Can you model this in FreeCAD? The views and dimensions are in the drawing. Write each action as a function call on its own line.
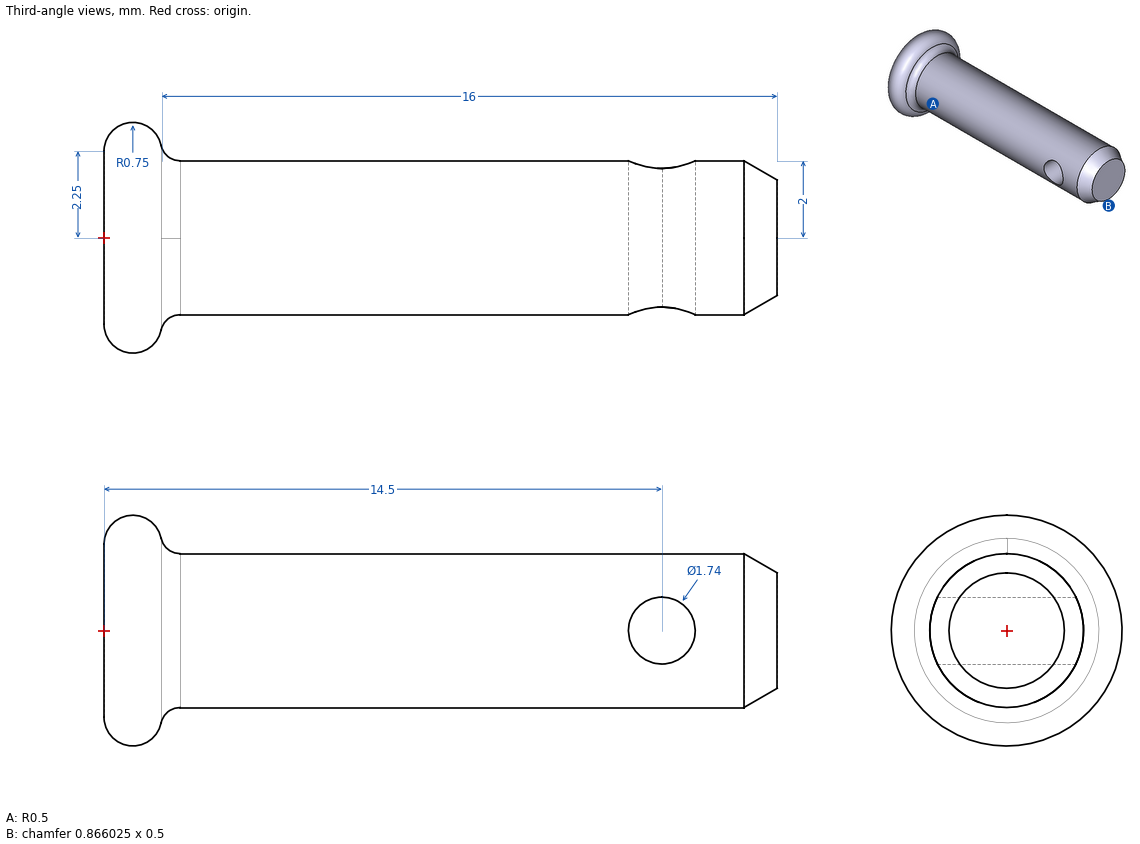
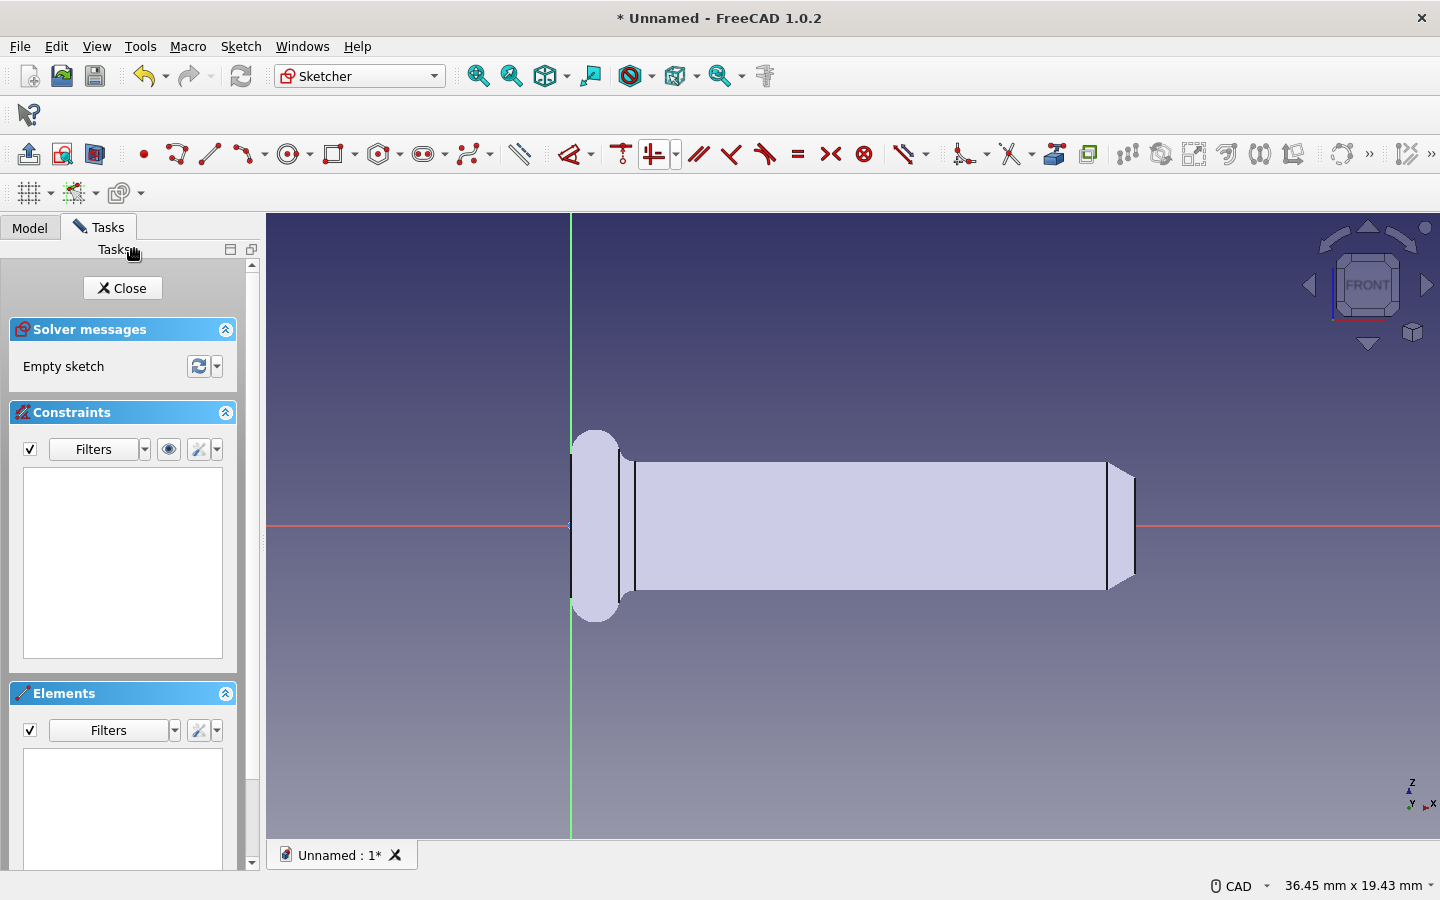
click(95, 154)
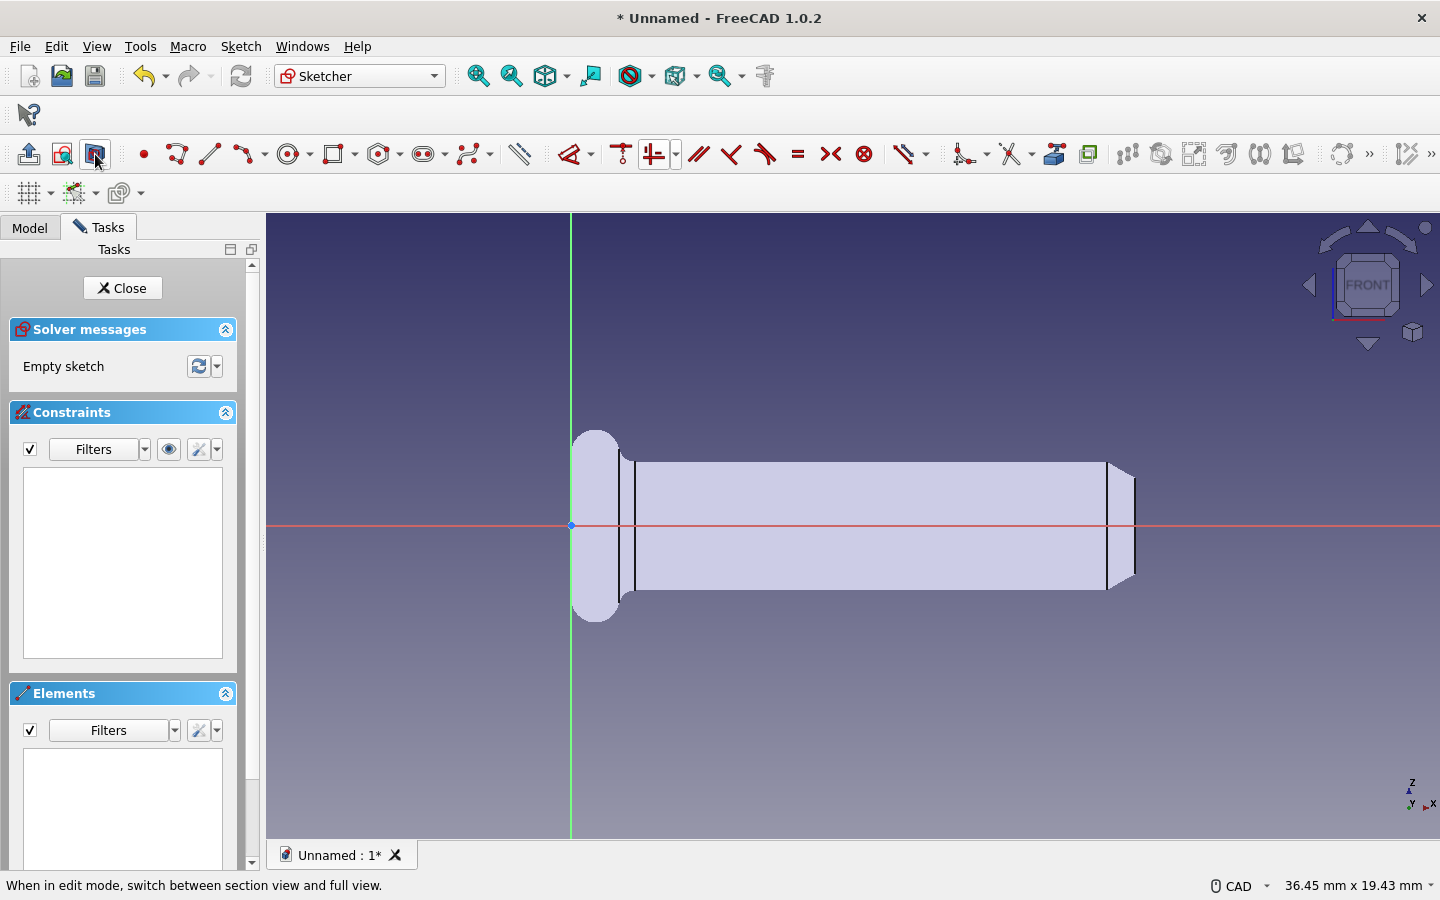
scroll(1078, 526, up, 10)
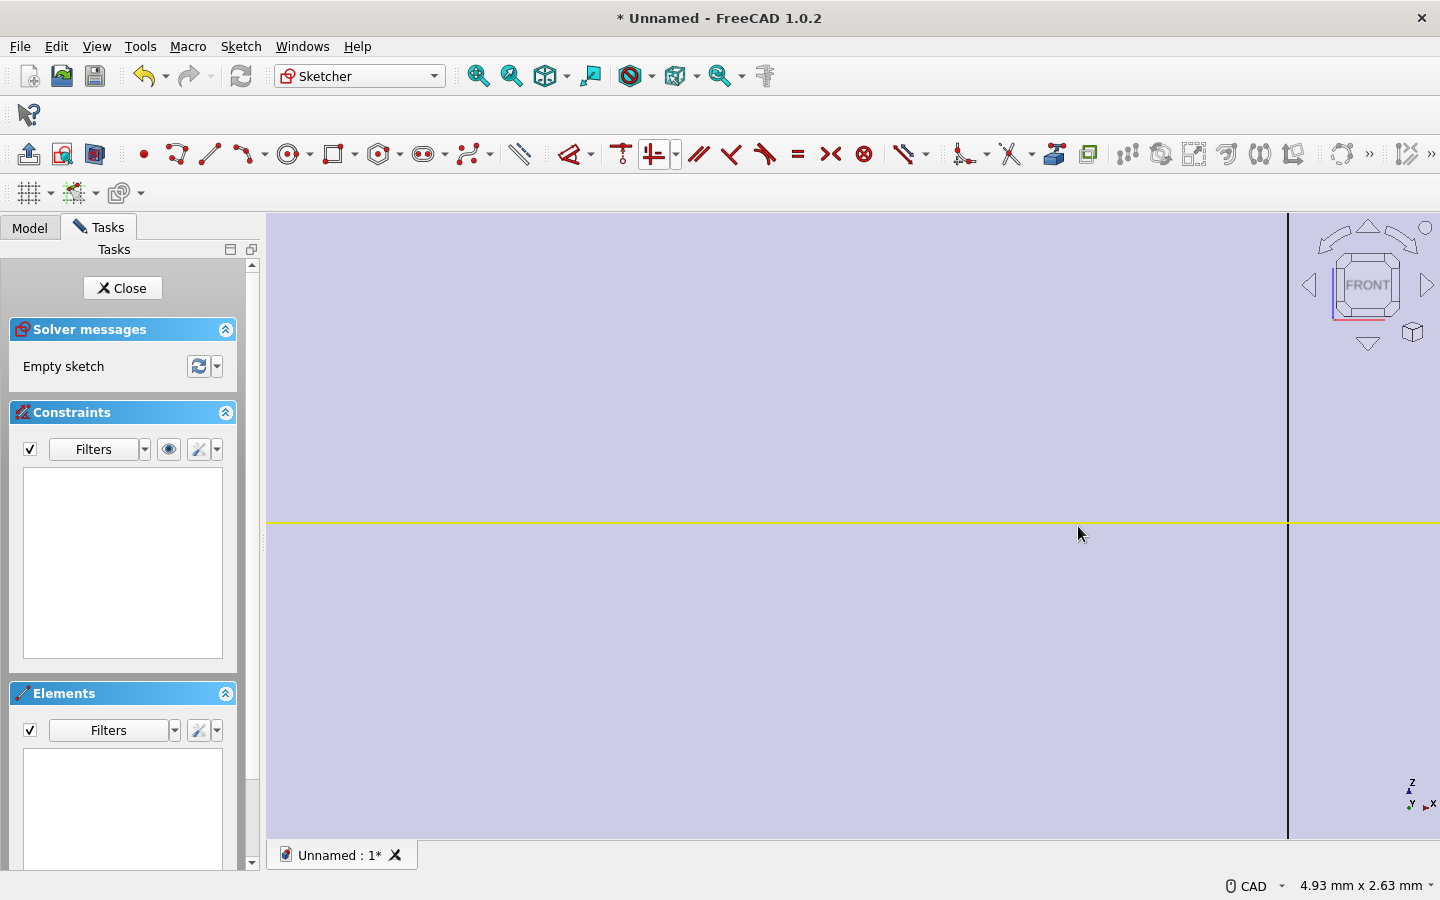
click(288, 154)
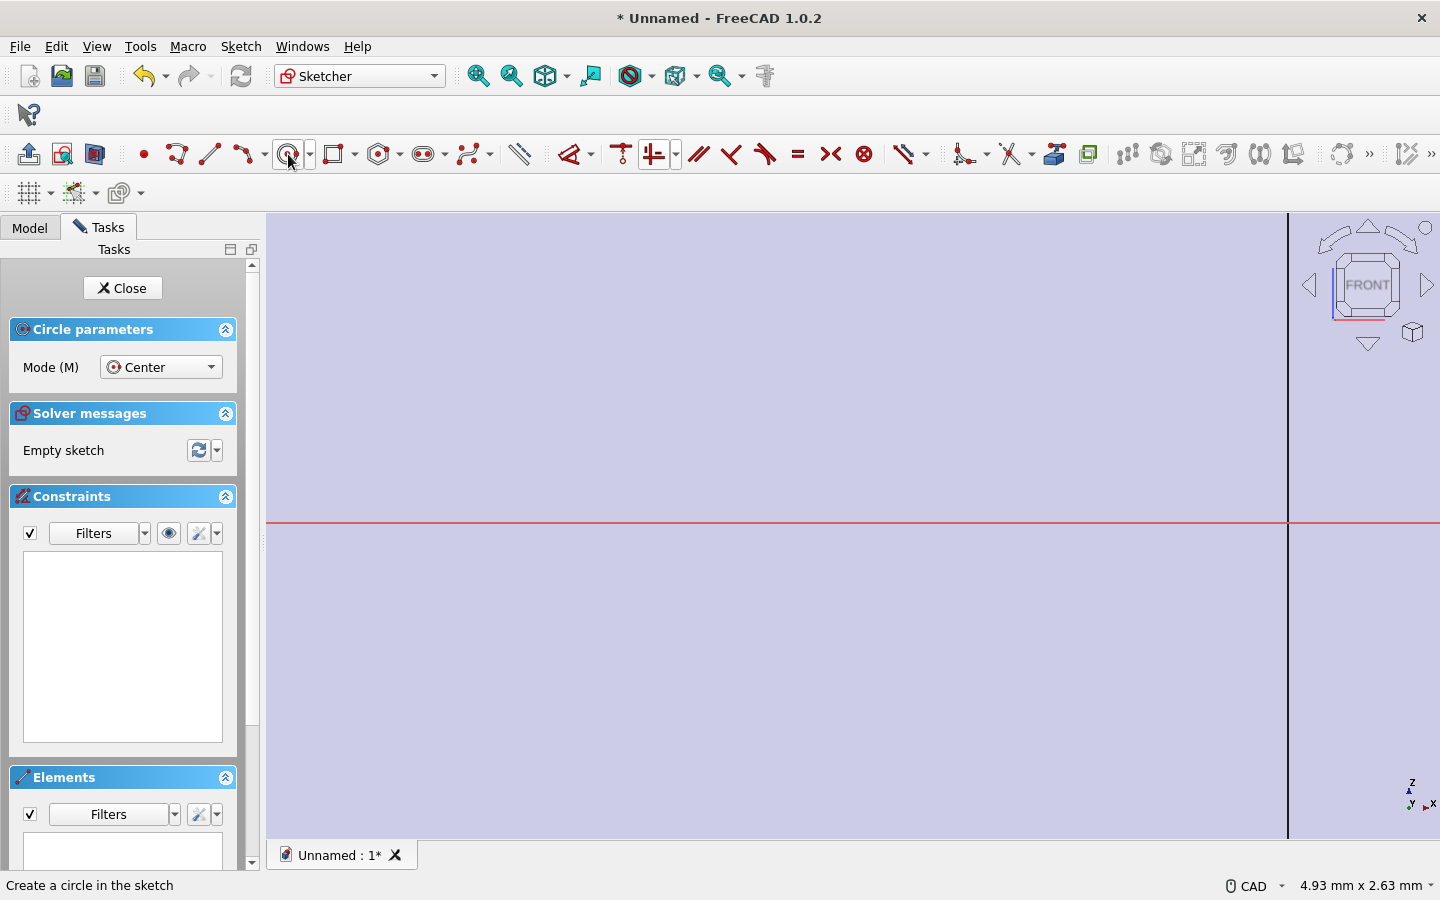
click(780, 523)
move(926, 376)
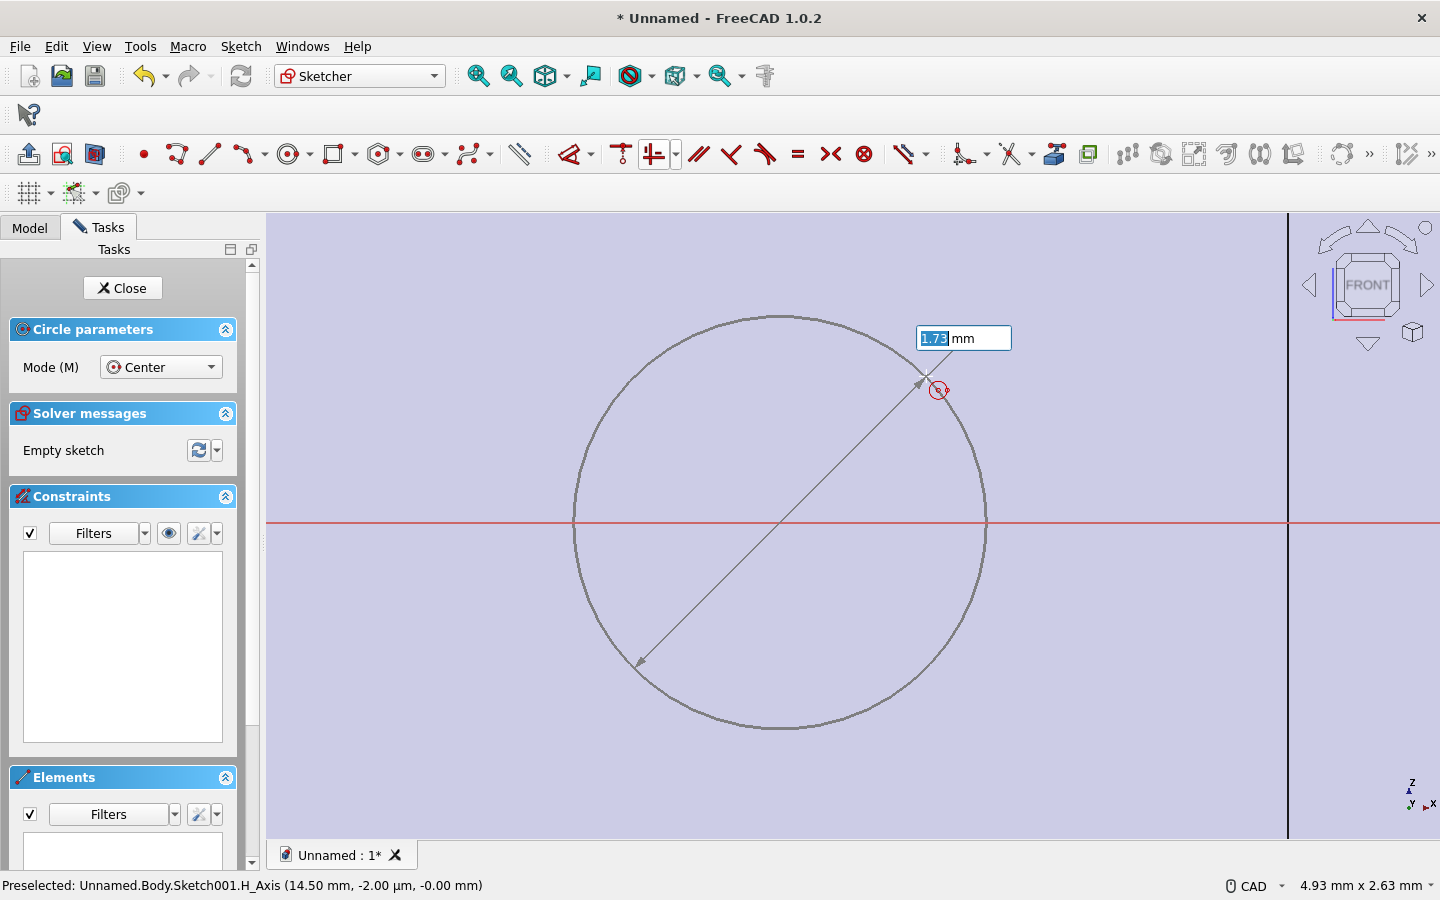
text(1.74)
key(Return)
key(Escape)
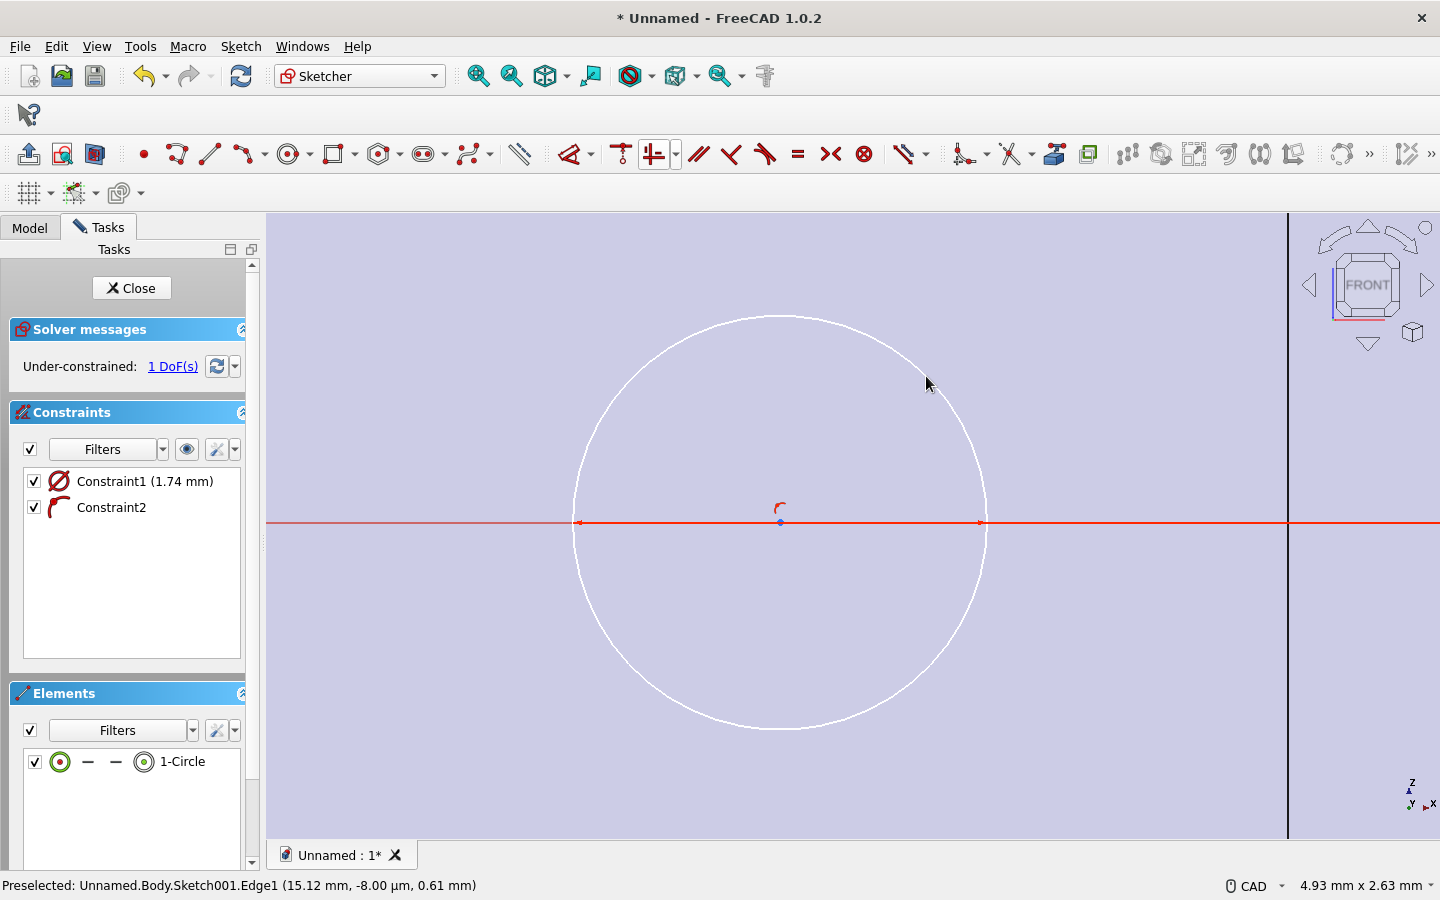
click(568, 154)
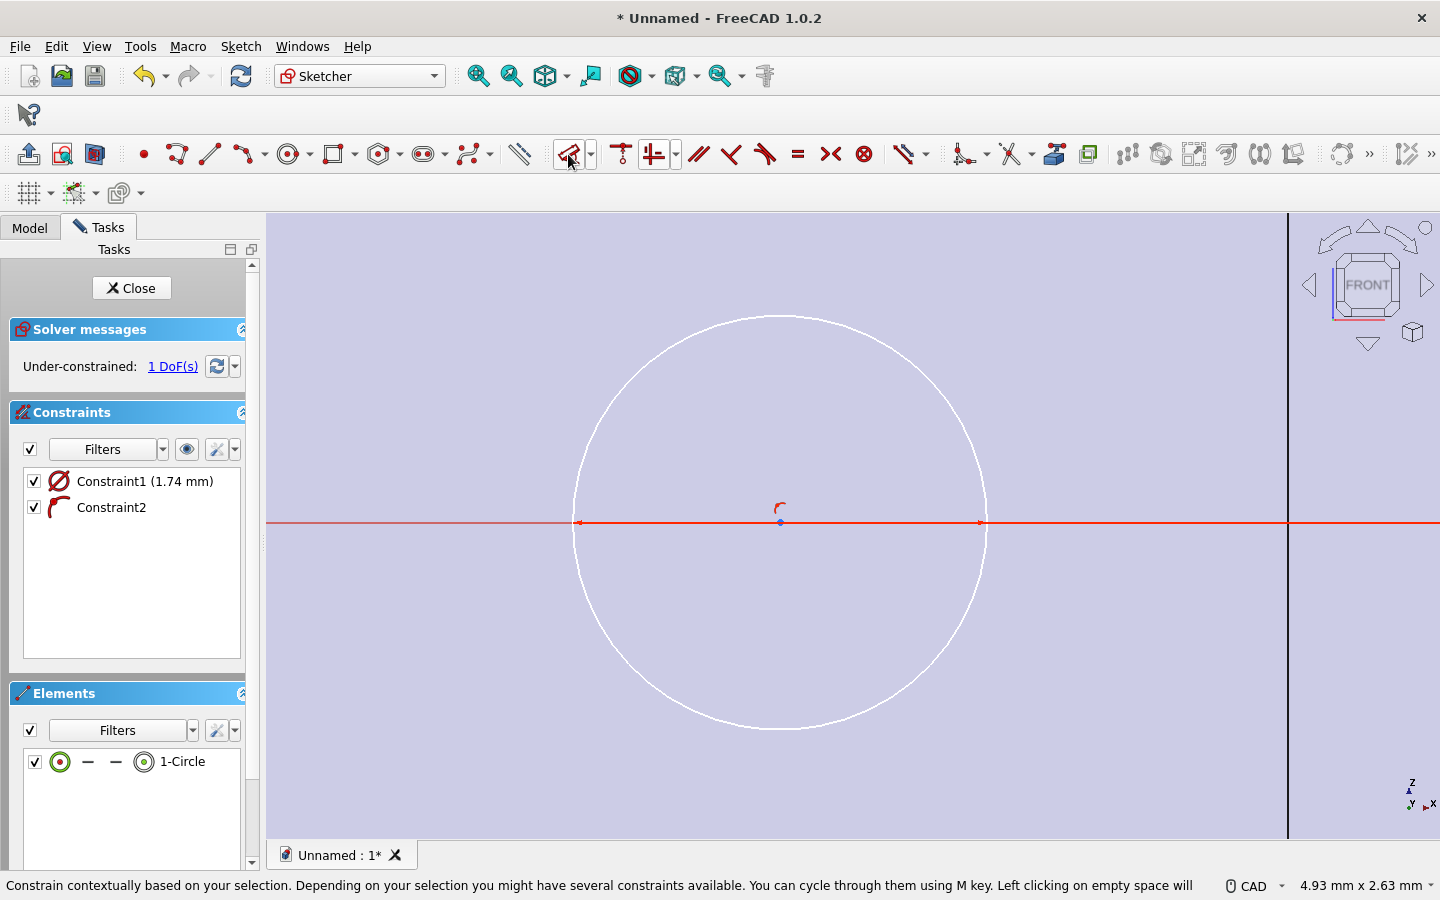
click(780, 523)
click(537, 557)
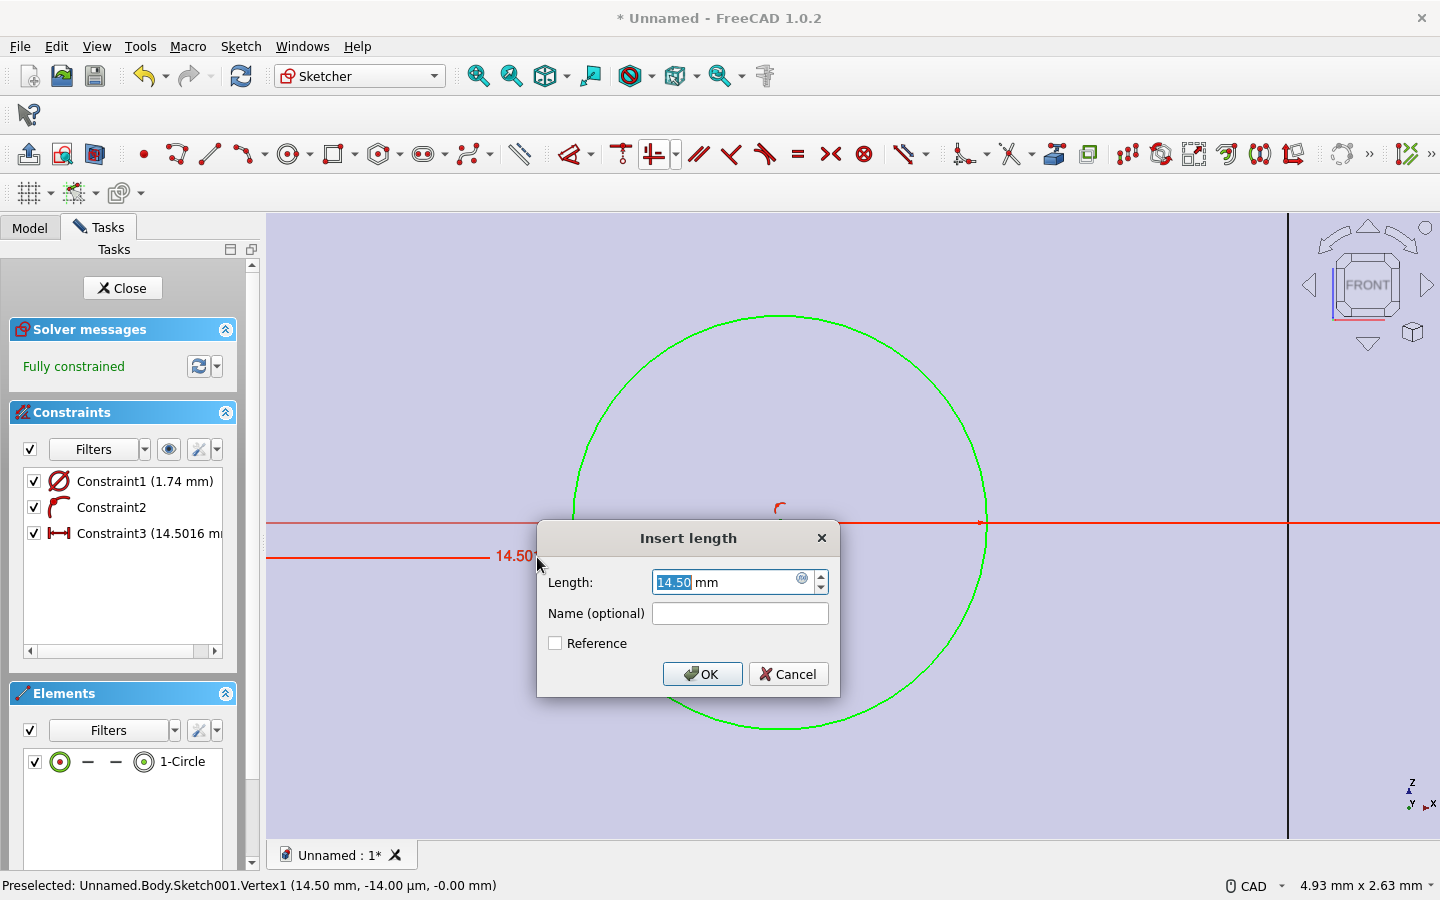
text(14.5)
key(Return)
key(Escape)